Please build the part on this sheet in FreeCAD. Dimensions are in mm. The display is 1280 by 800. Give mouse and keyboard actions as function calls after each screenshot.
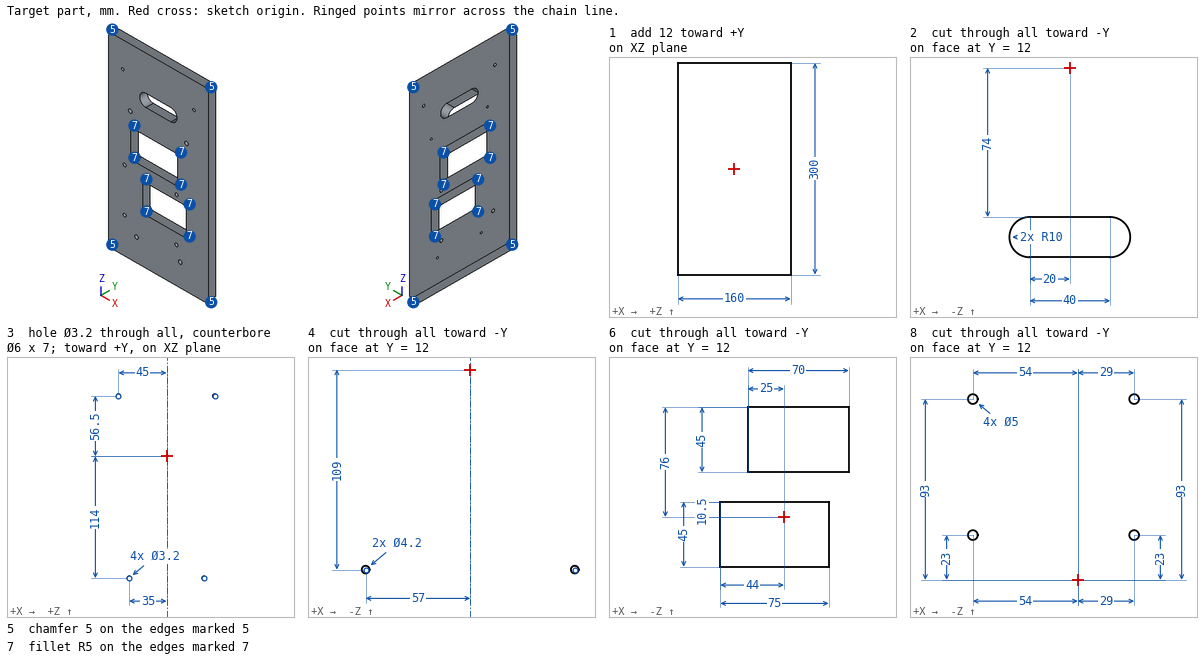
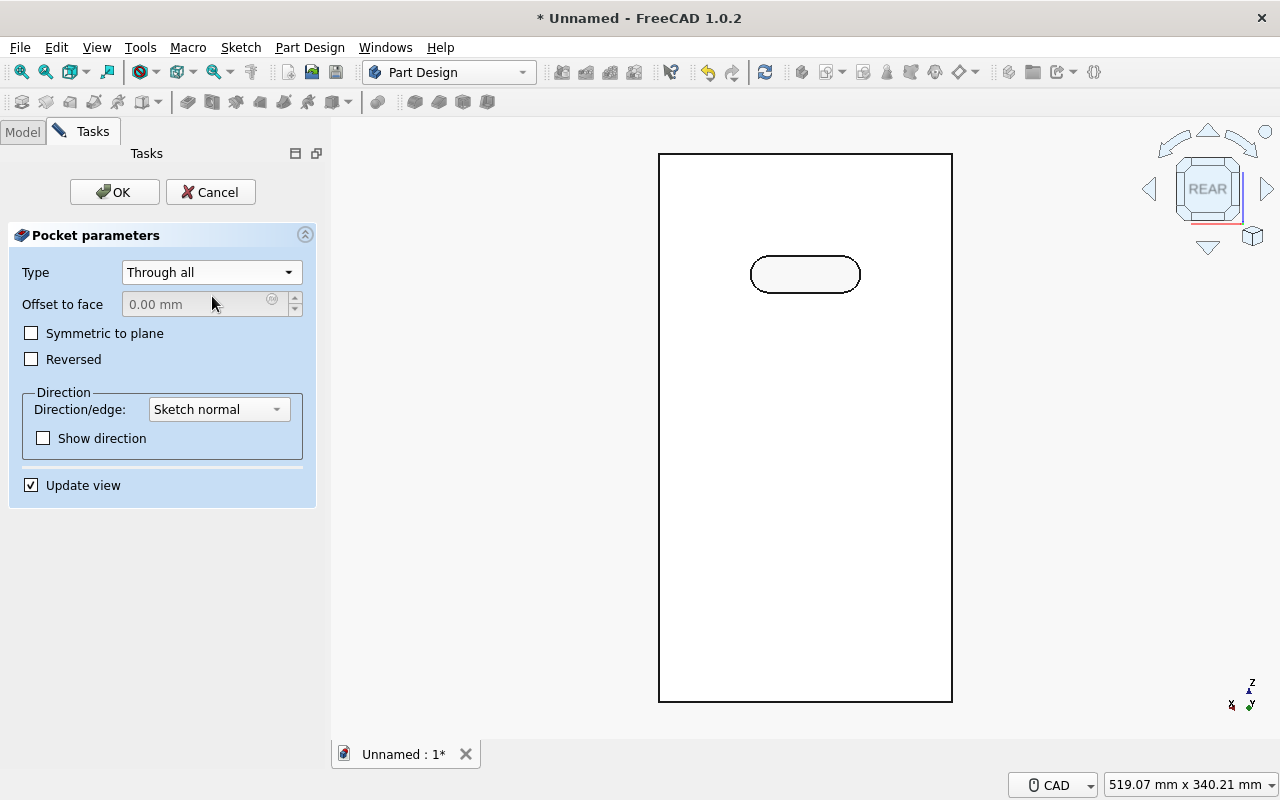
click(115, 192)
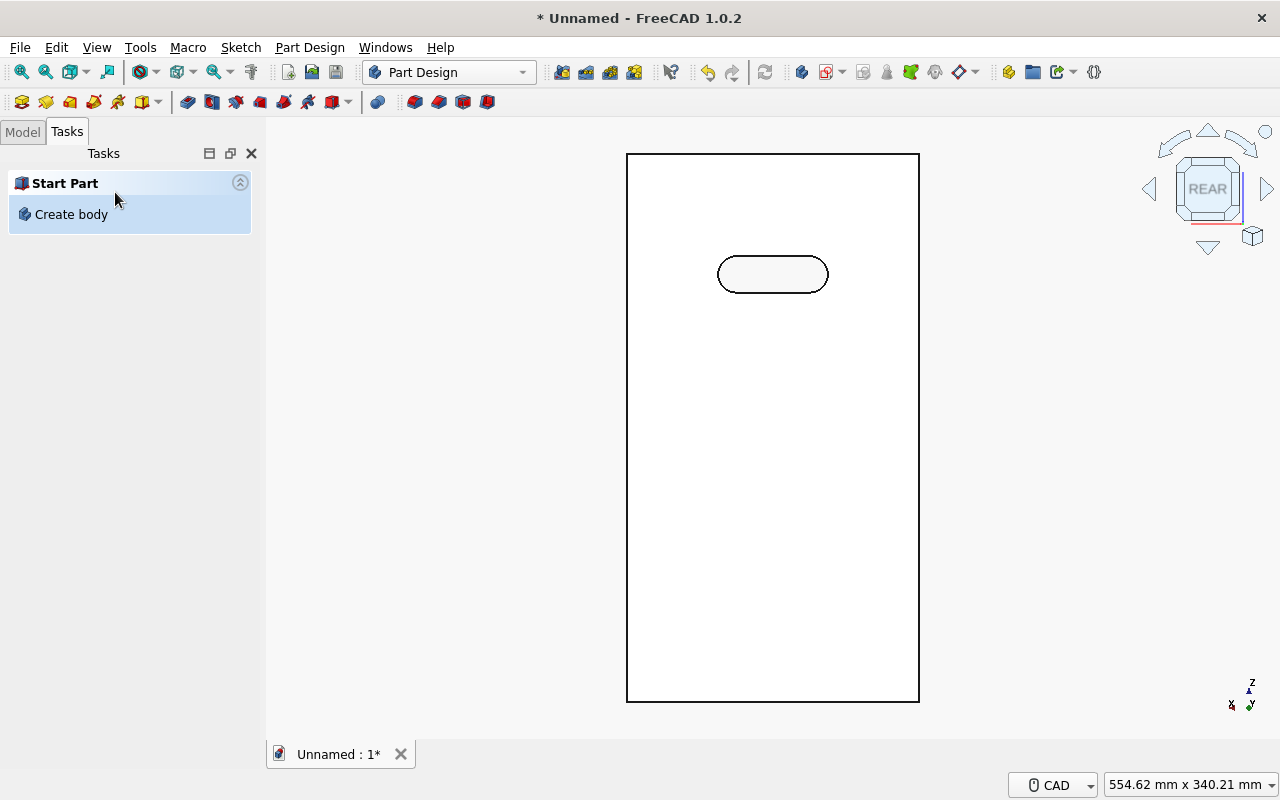
click(826, 72)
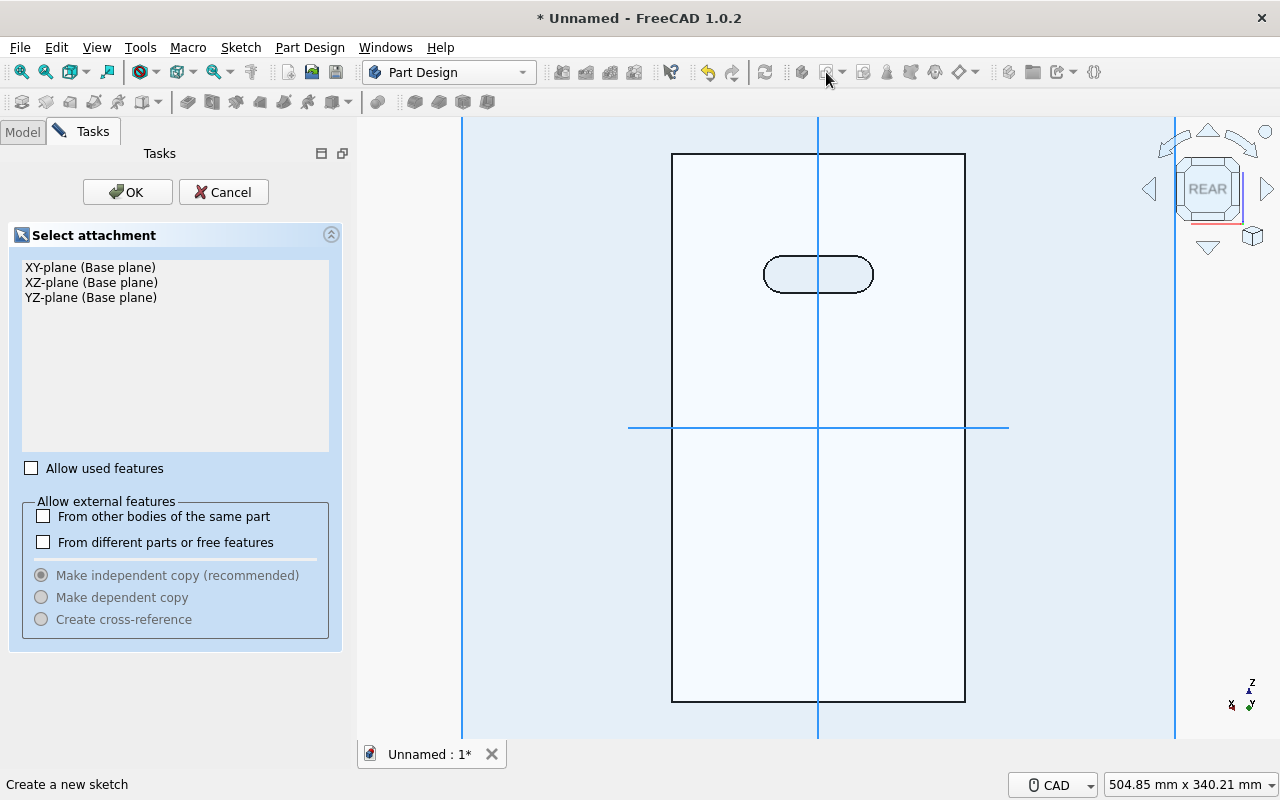
click(82, 282)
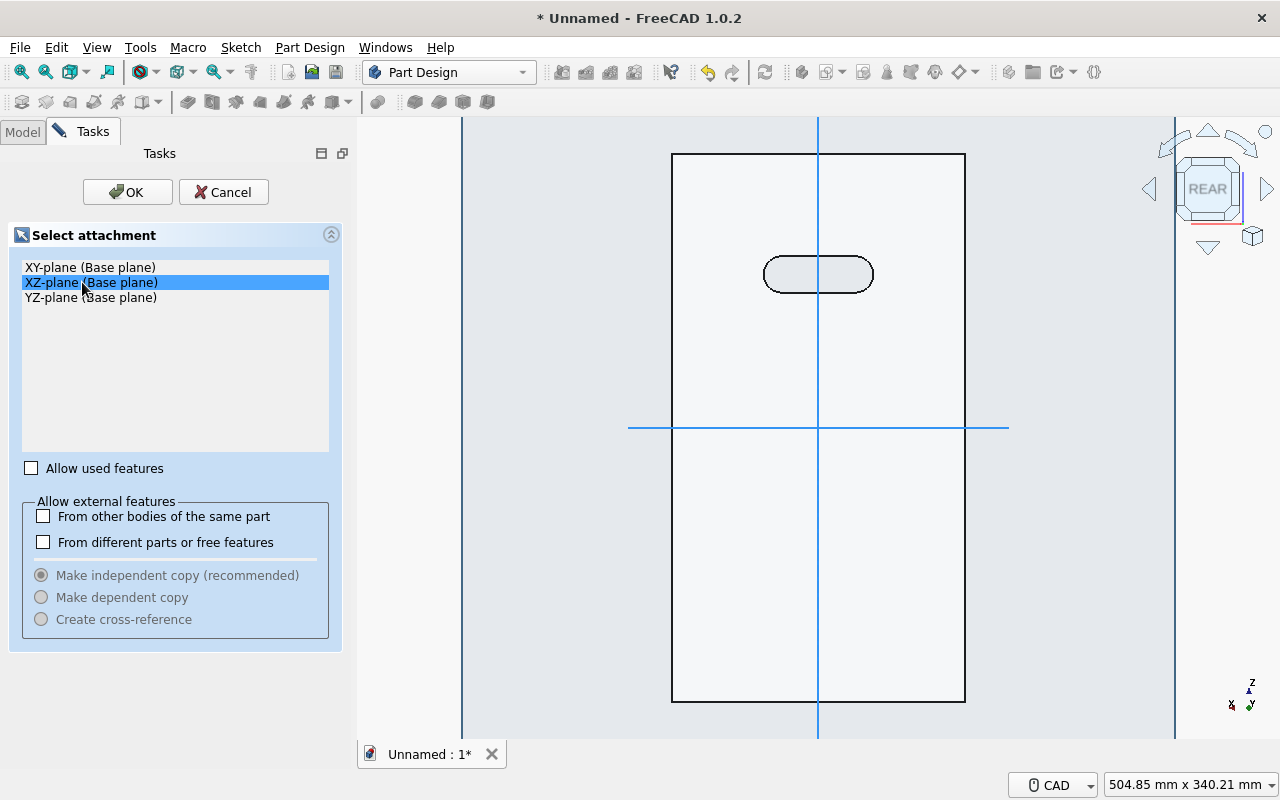
click(128, 192)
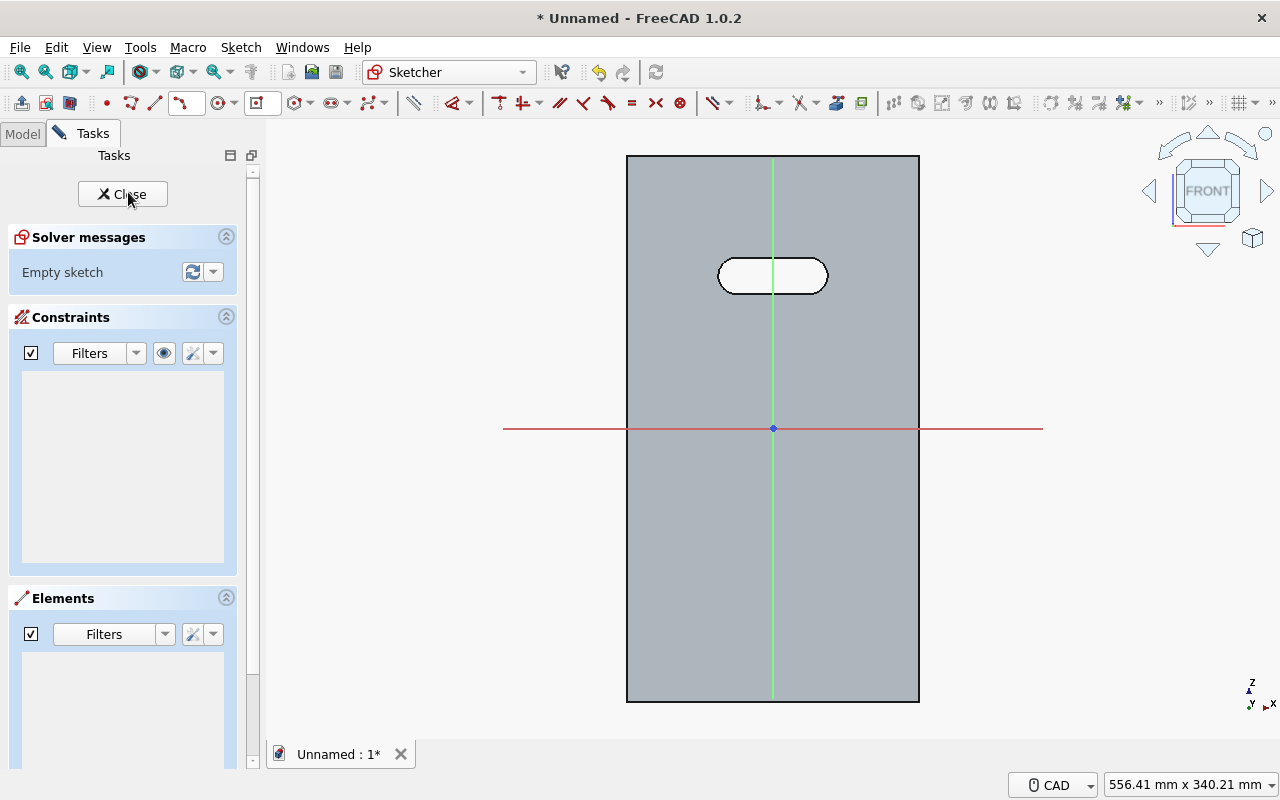
click(218, 104)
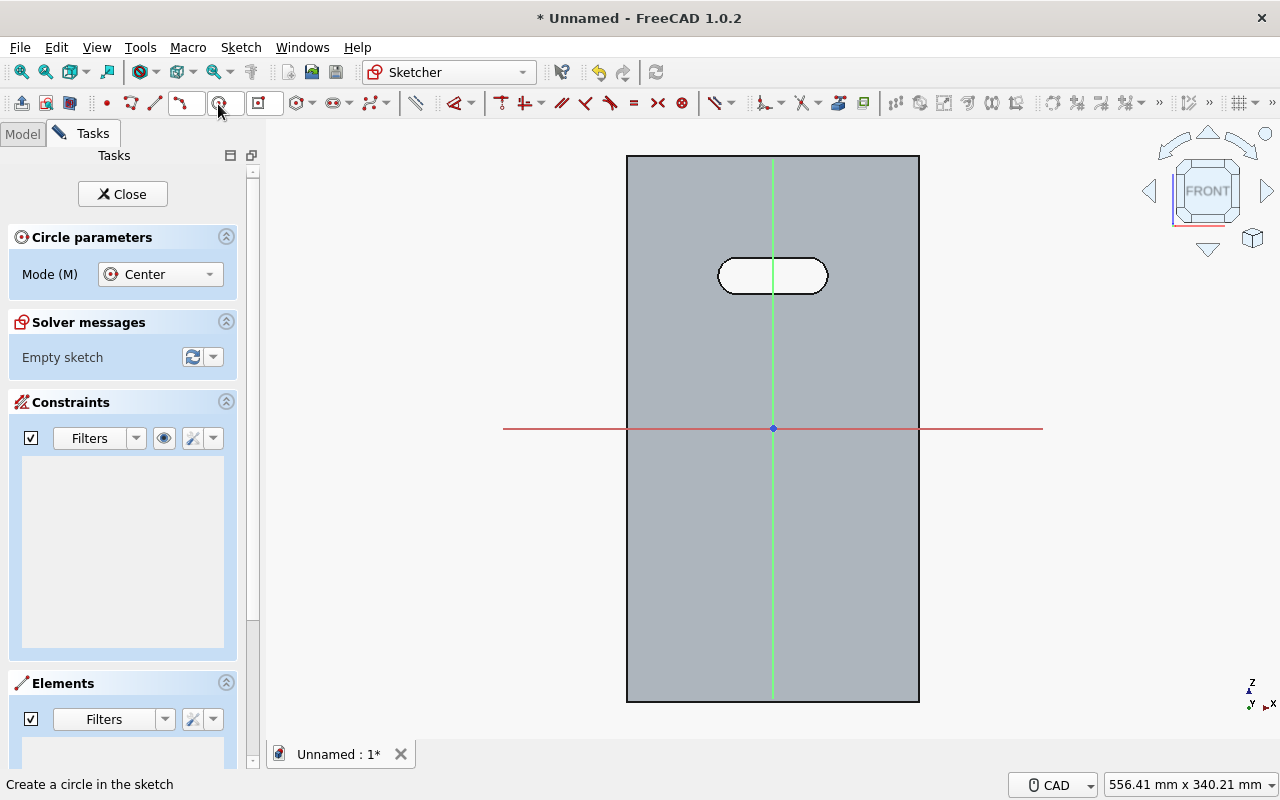
scroll(709, 637, up, 11)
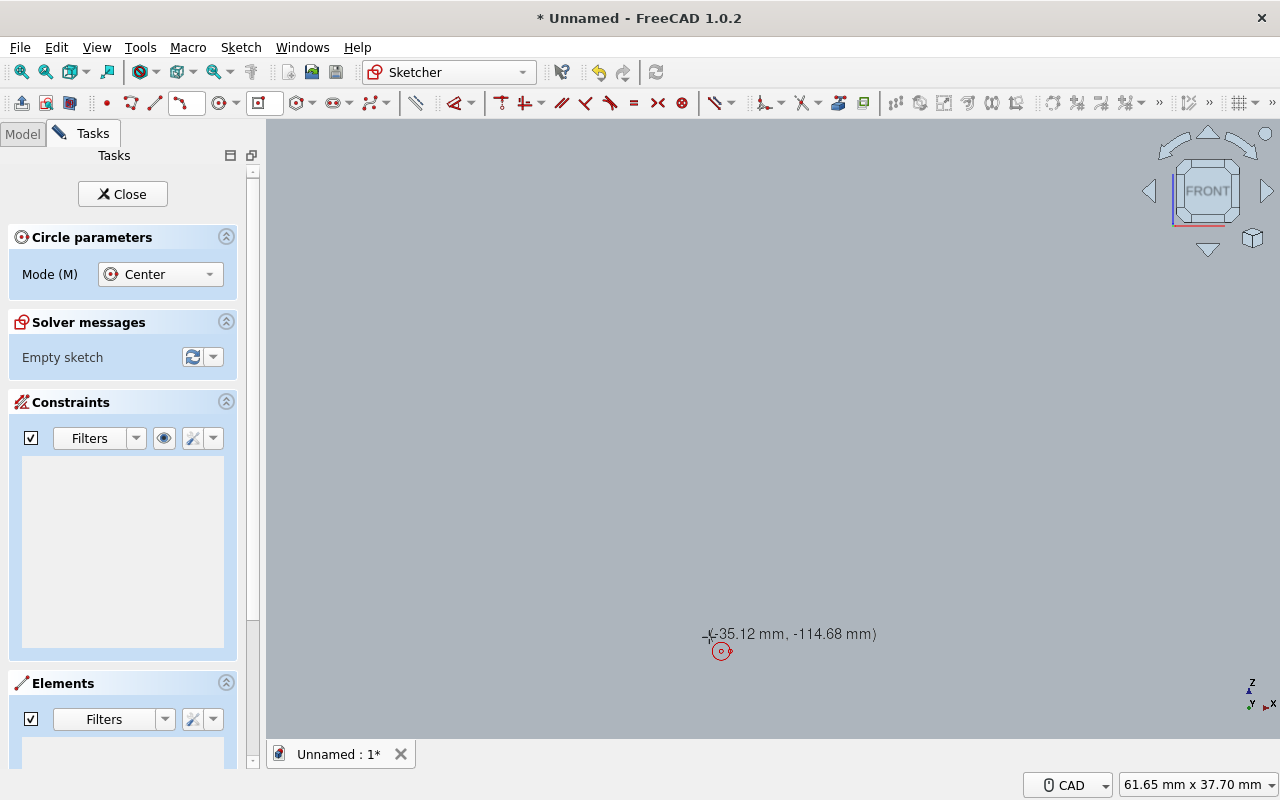
scroll(614, 617, down, 10)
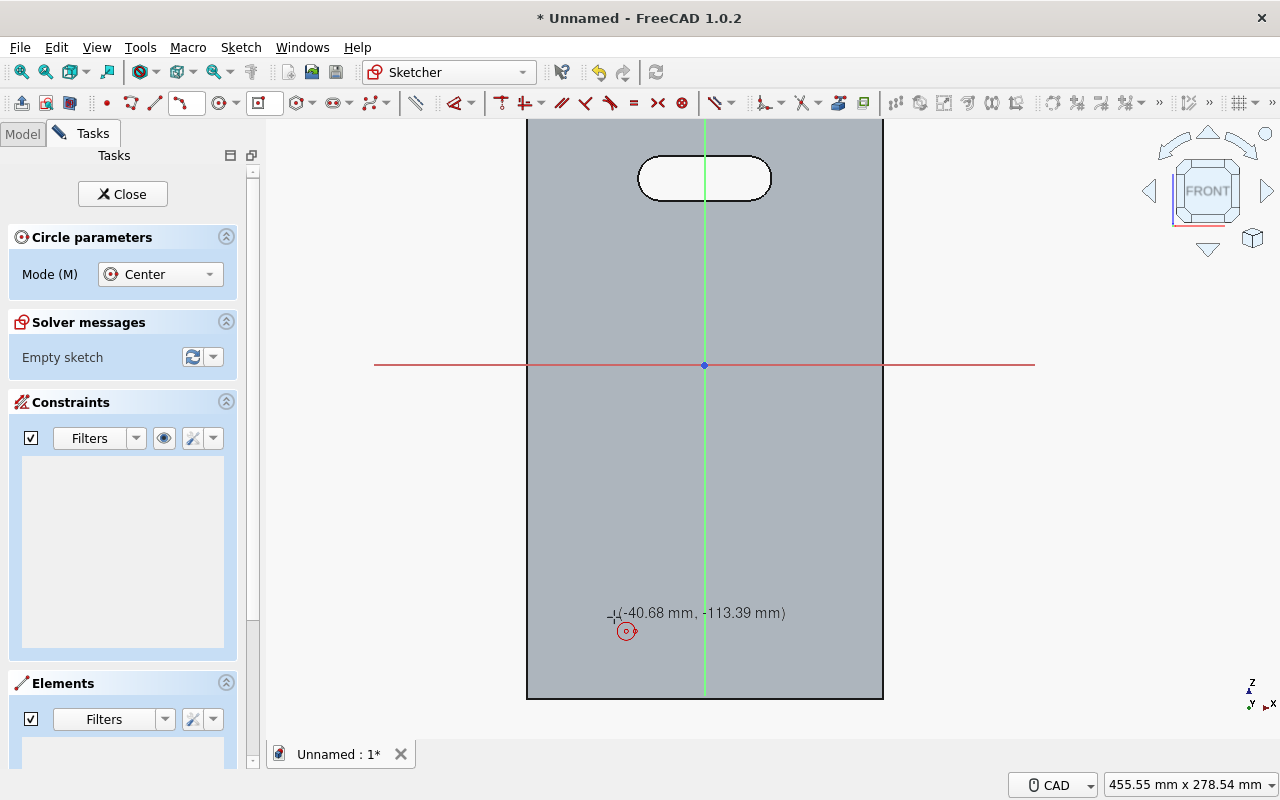
click(627, 619)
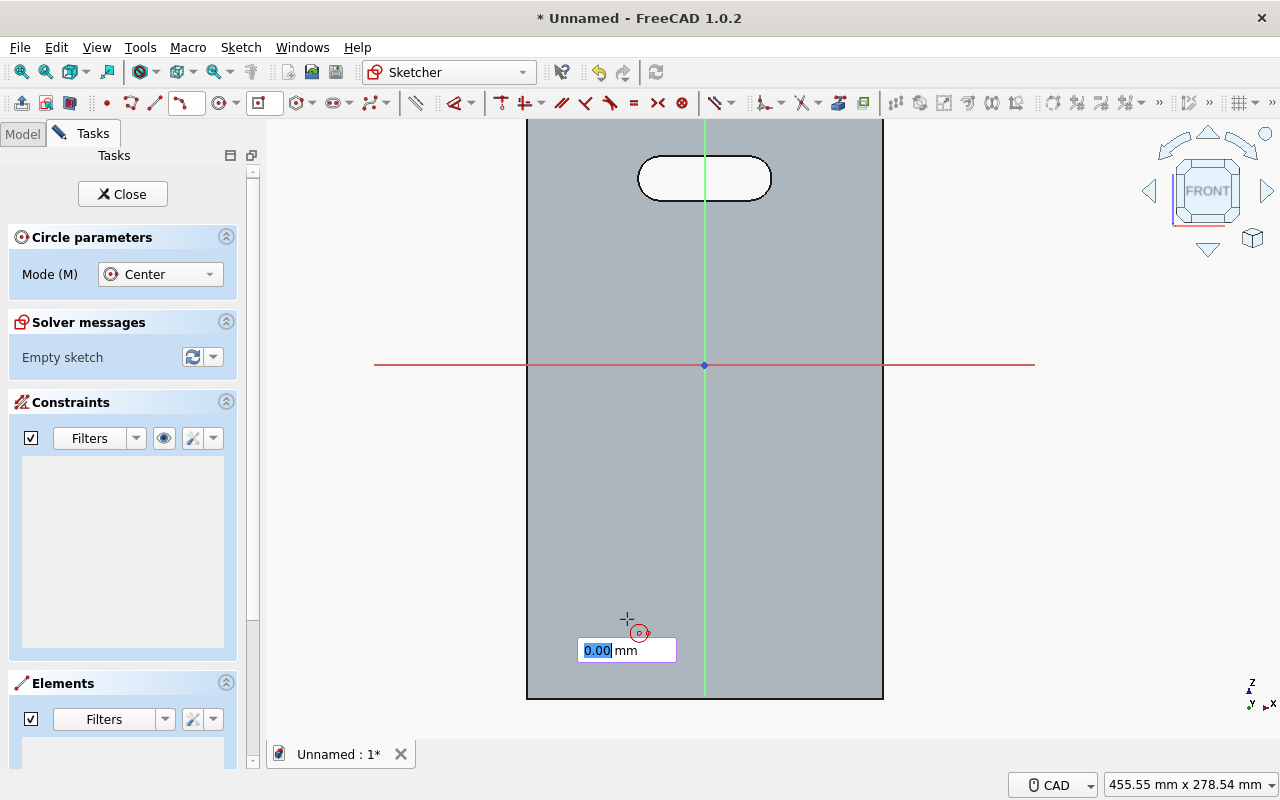
scroll(629, 617, up, 8)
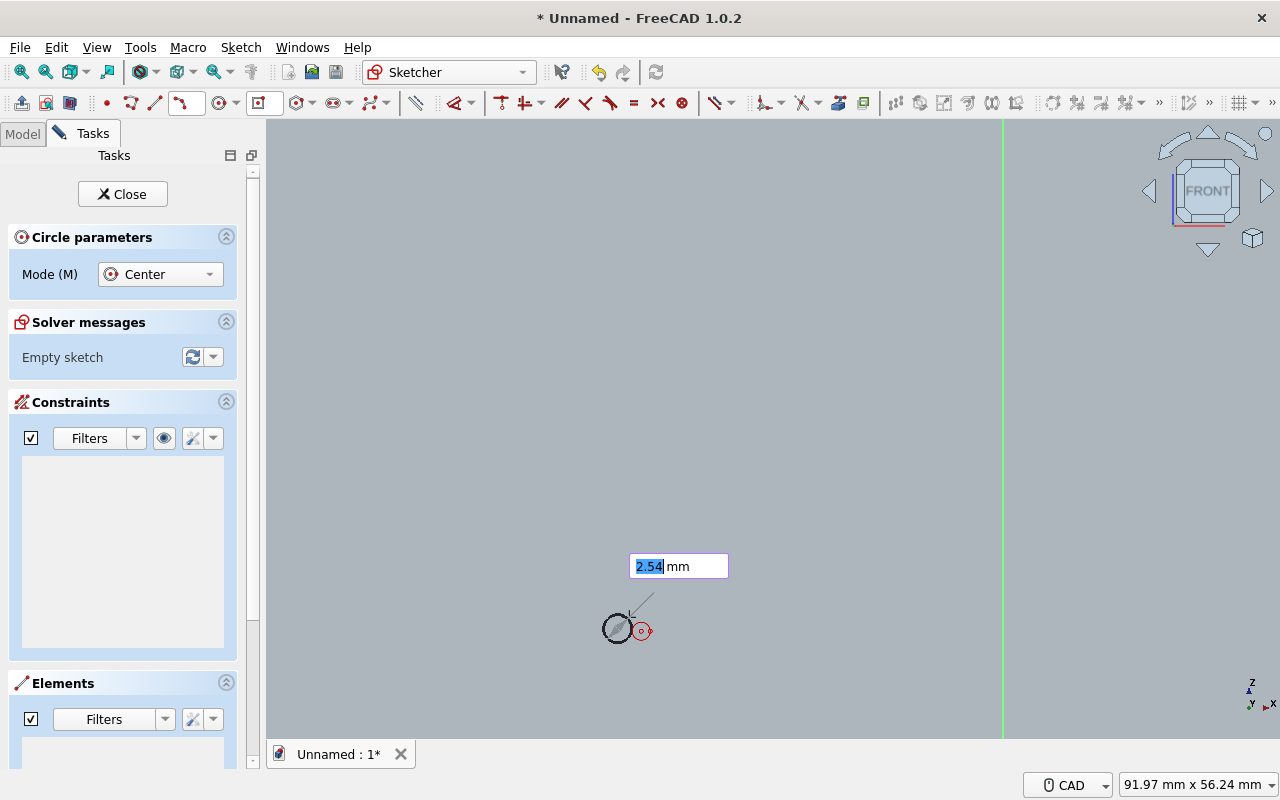
click(630, 612)